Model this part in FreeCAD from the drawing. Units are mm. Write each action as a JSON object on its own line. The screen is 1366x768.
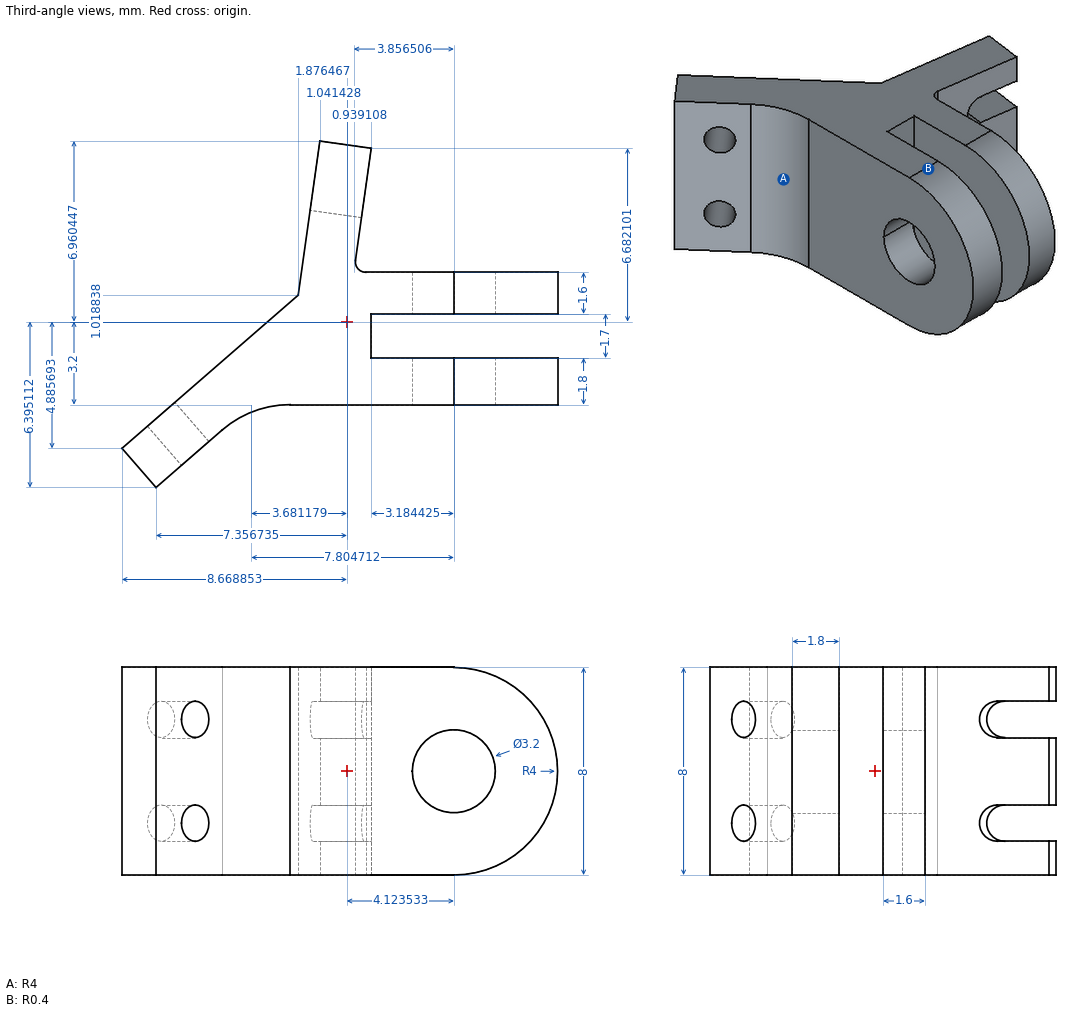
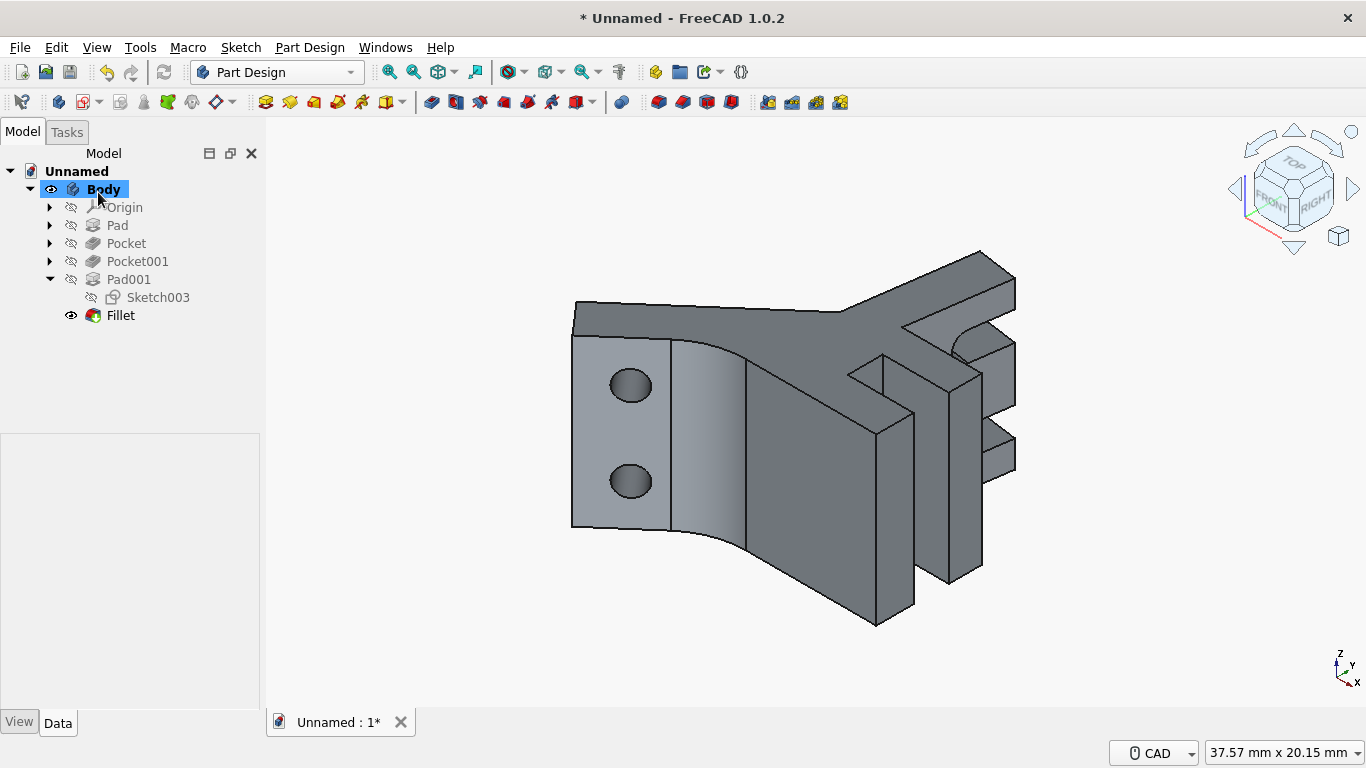
{"action": "key", "text": "1"}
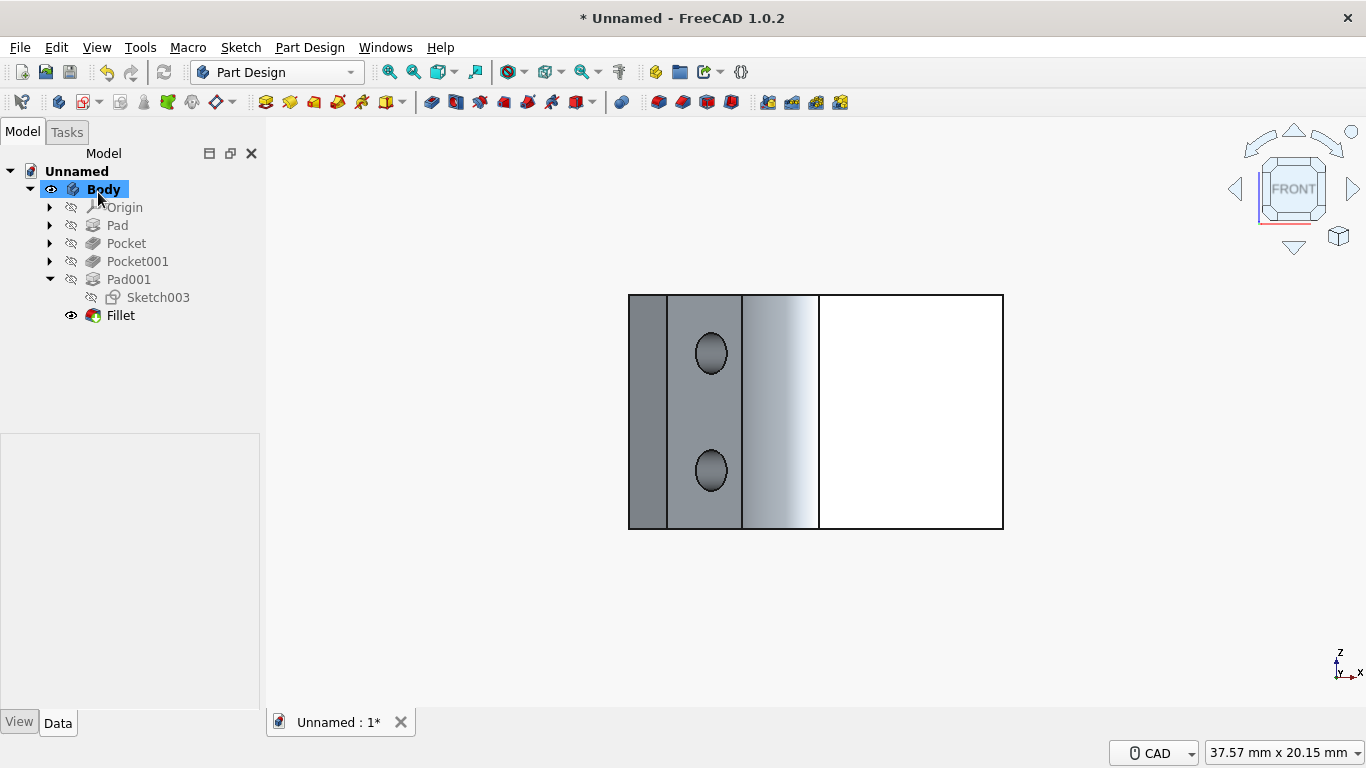
{"action": "left_click", "coordinate": [390, 72]}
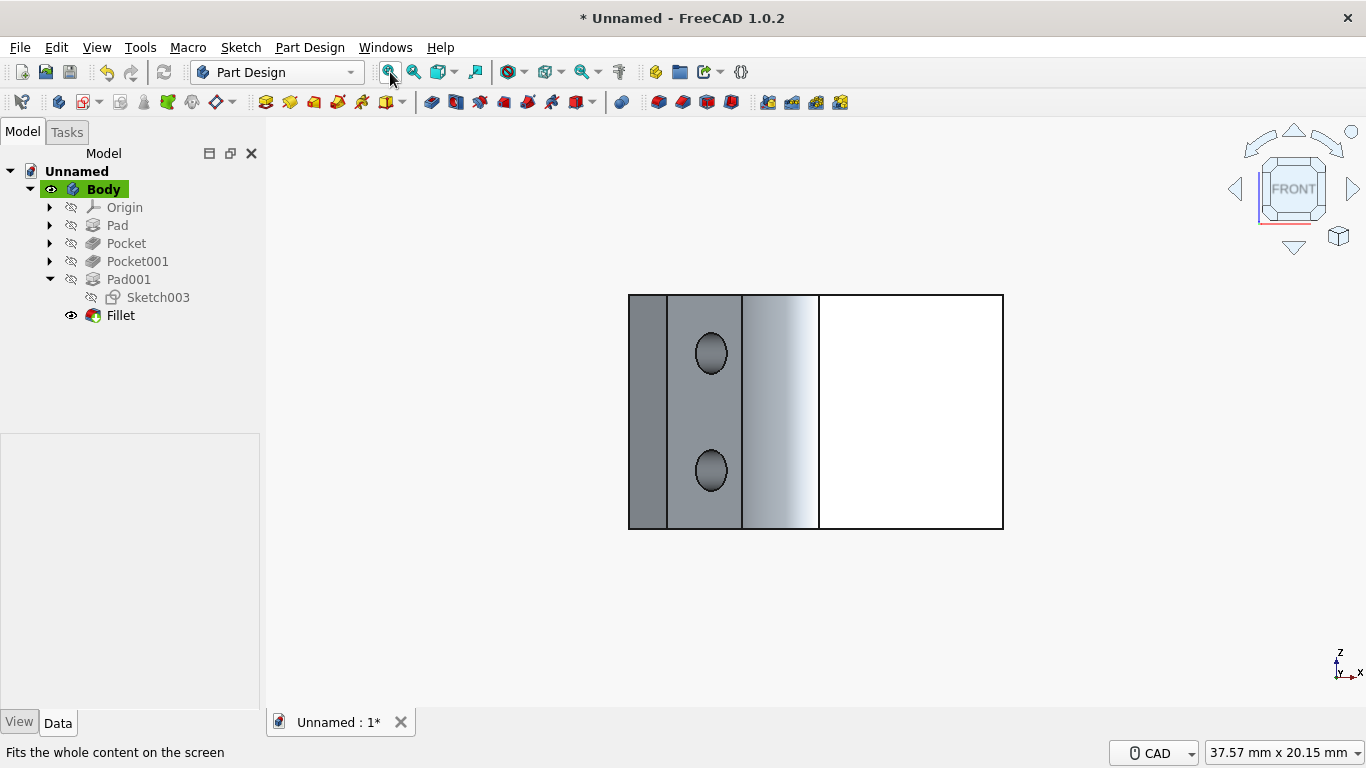
{"action": "key", "text": "3"}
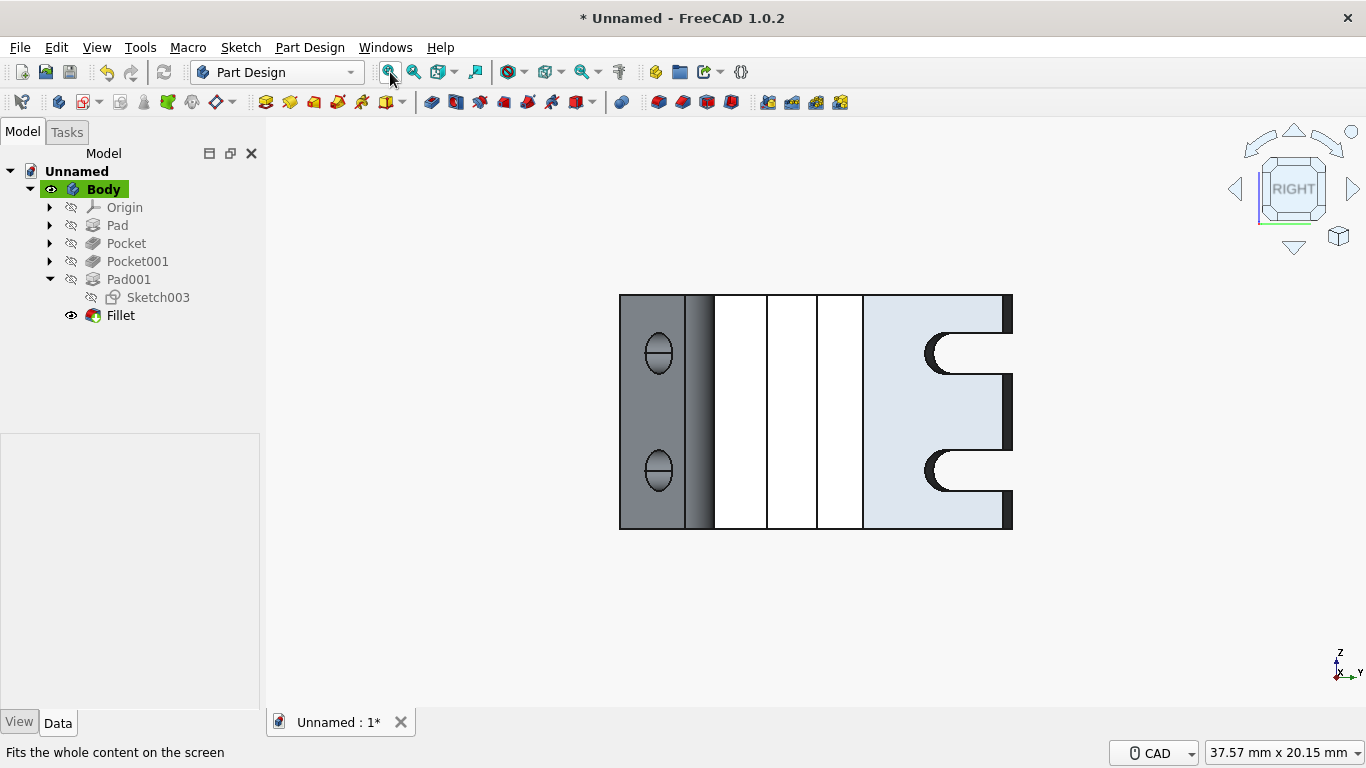
{"action": "left_click", "coordinate": [390, 72]}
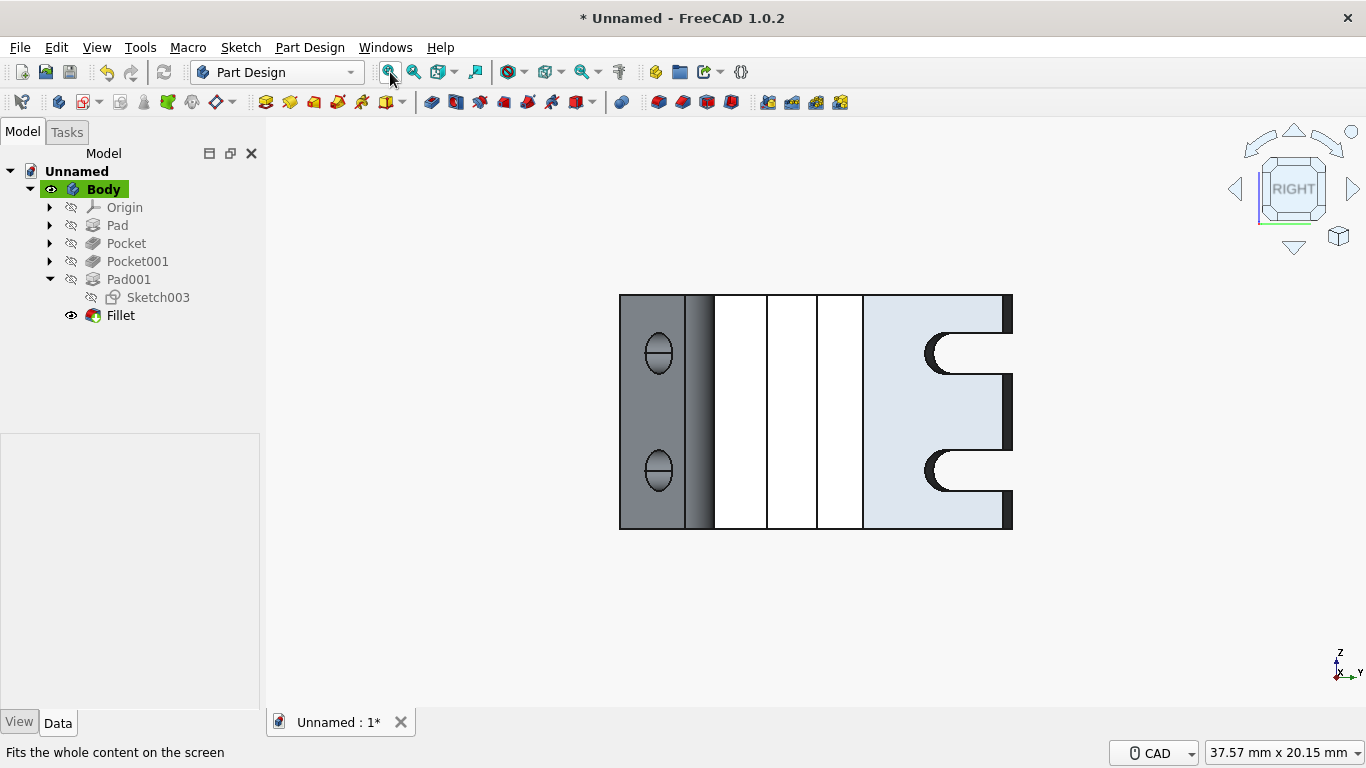
{"action": "key", "text": "5"}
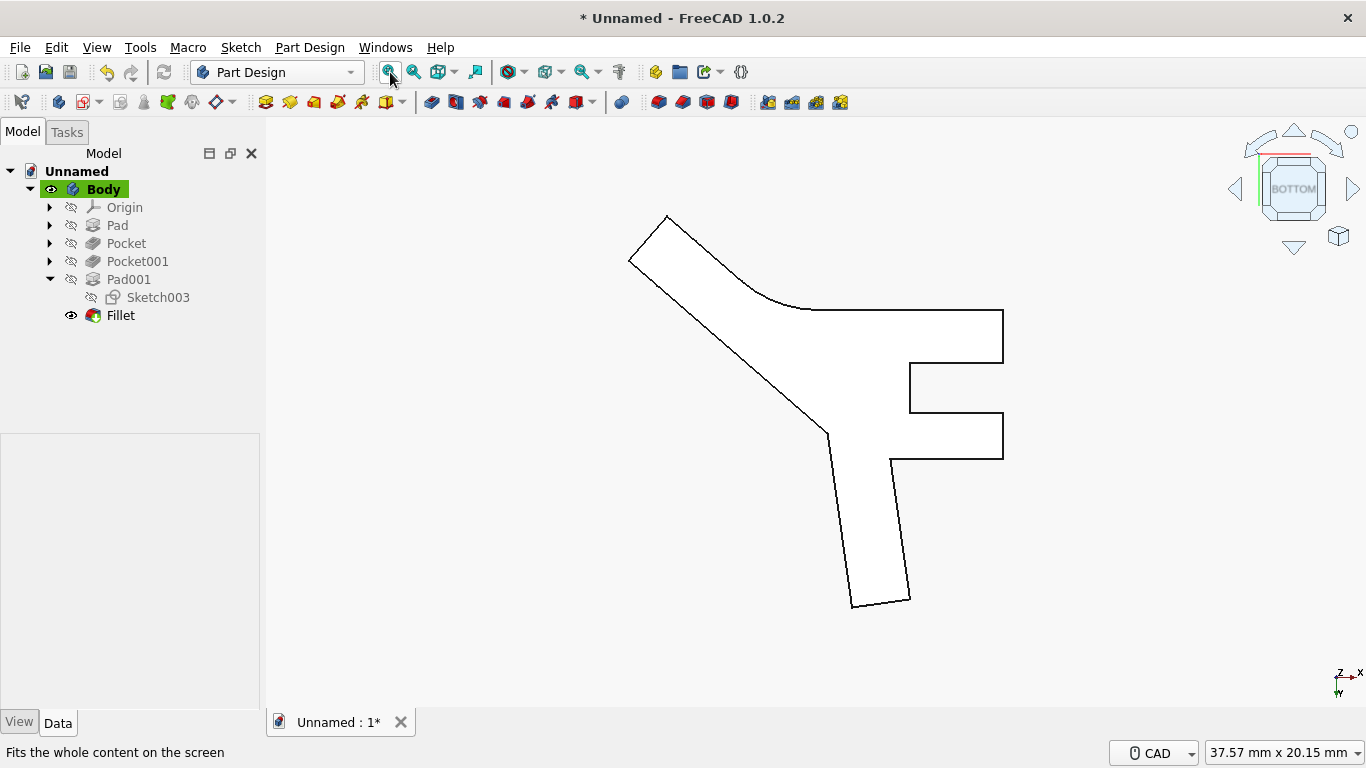
{"action": "key", "text": "4"}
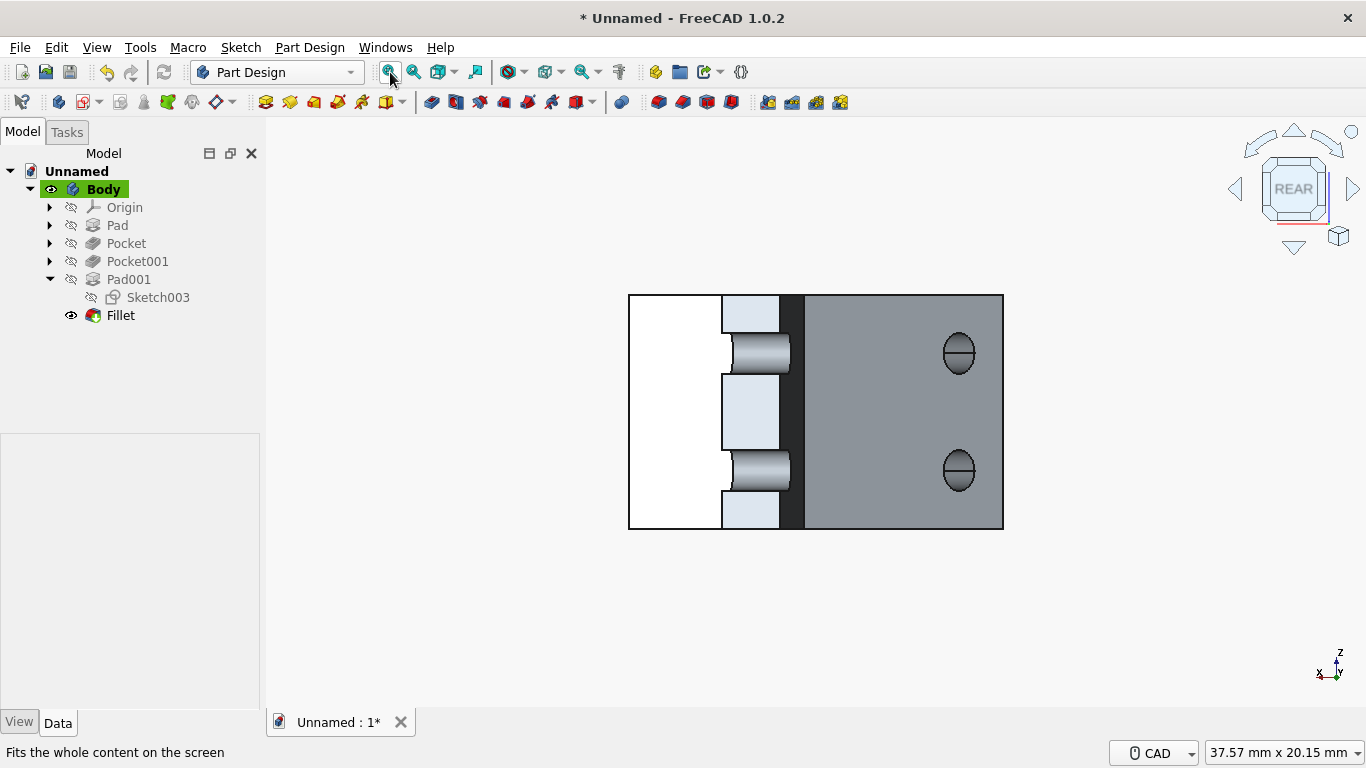
{"action": "left_click", "coordinate": [390, 72]}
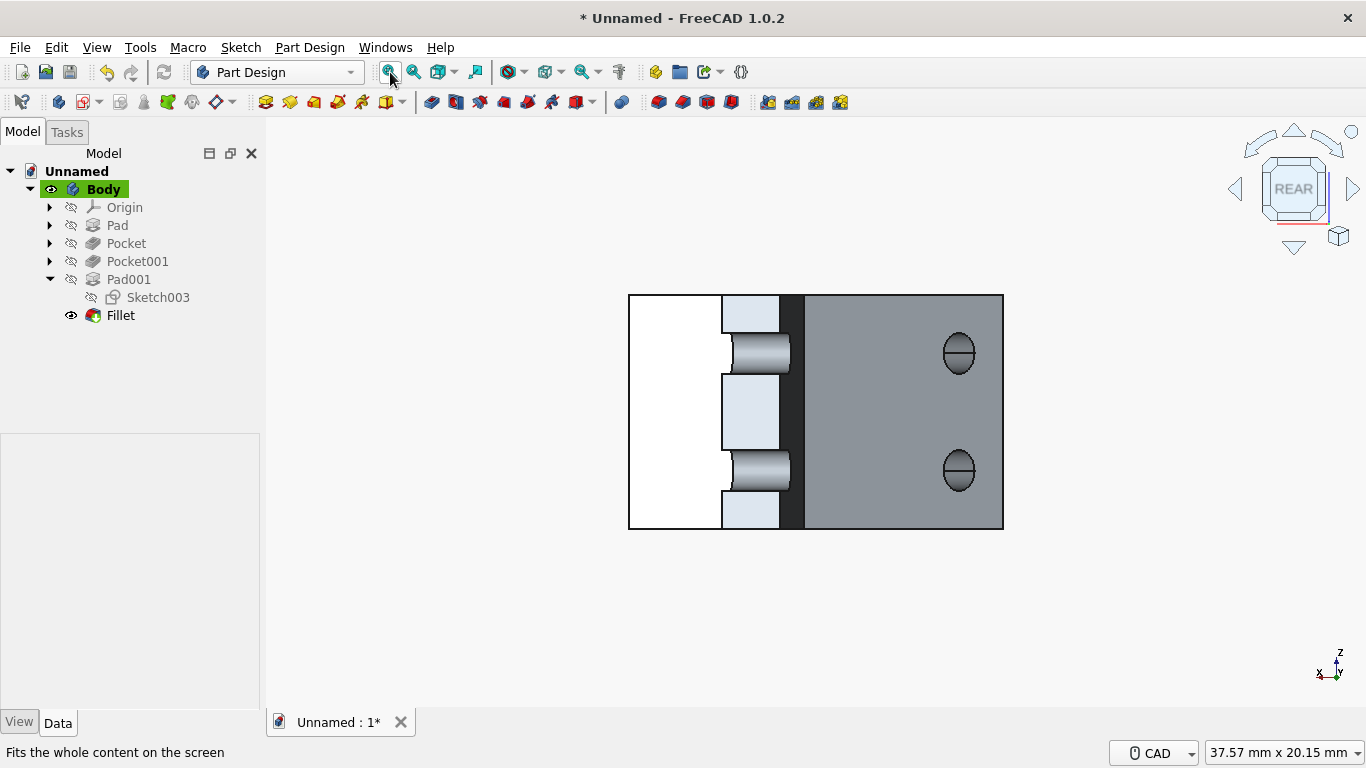
{"action": "key", "text": "6"}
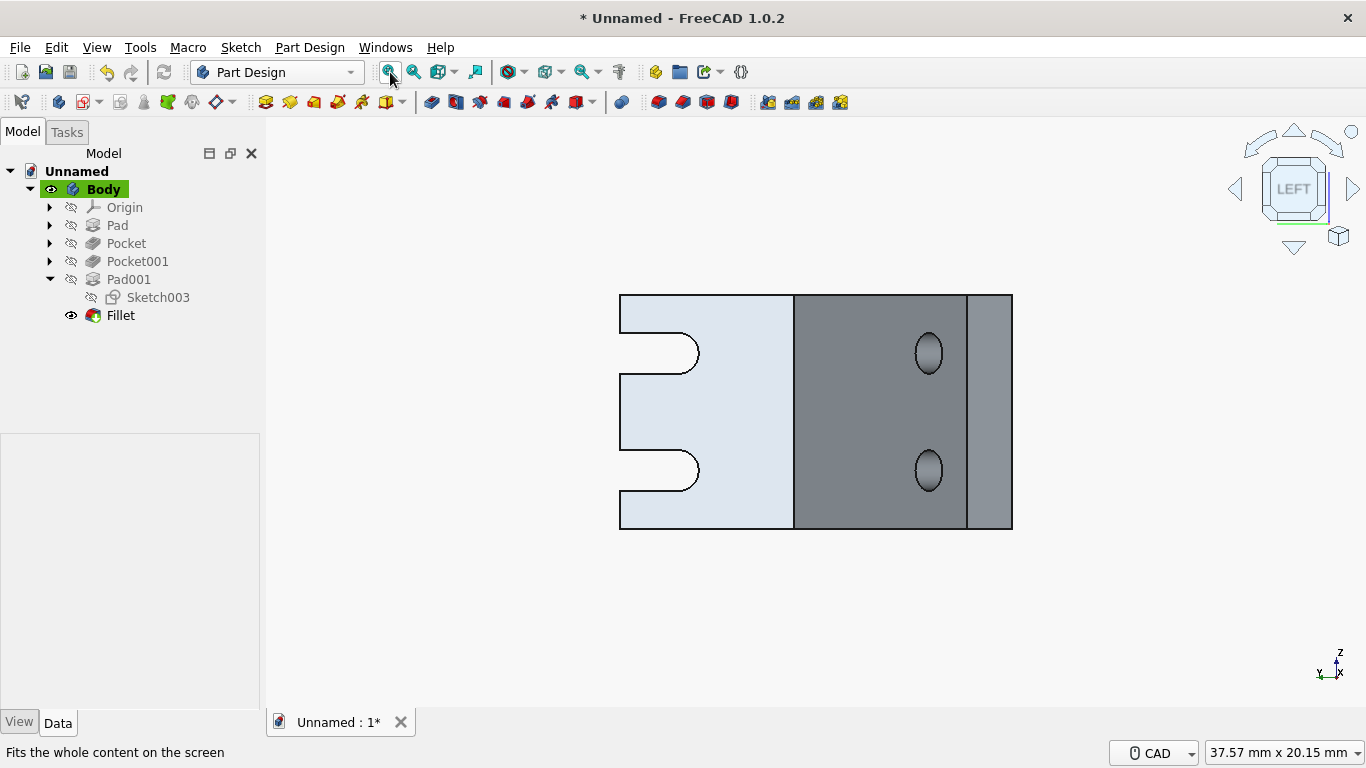
{"action": "left_click", "coordinate": [390, 72]}